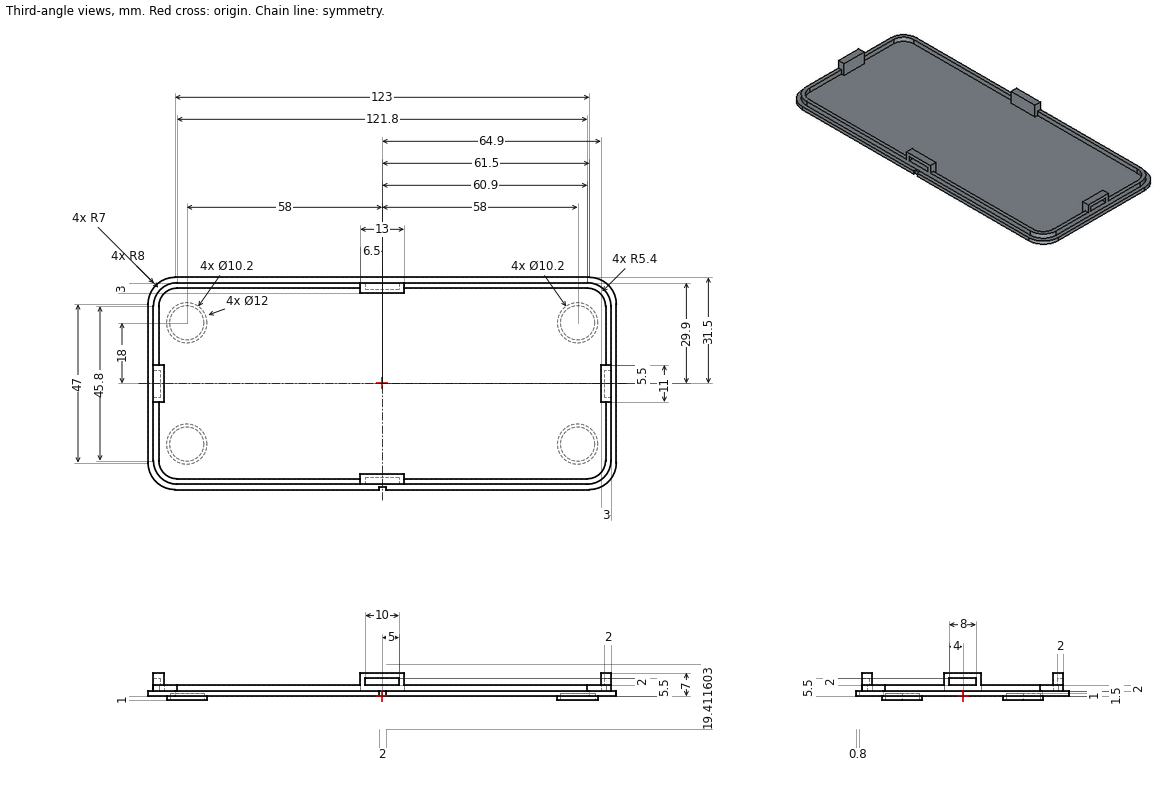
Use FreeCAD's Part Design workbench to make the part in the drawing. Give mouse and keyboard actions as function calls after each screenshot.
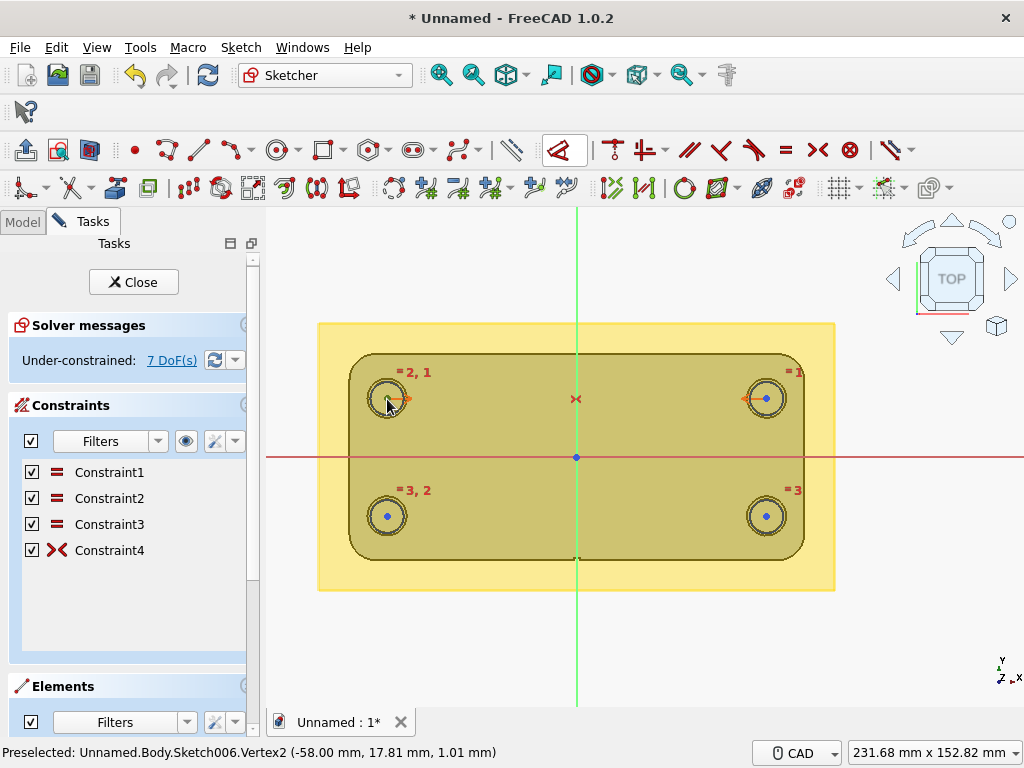
click(387, 517)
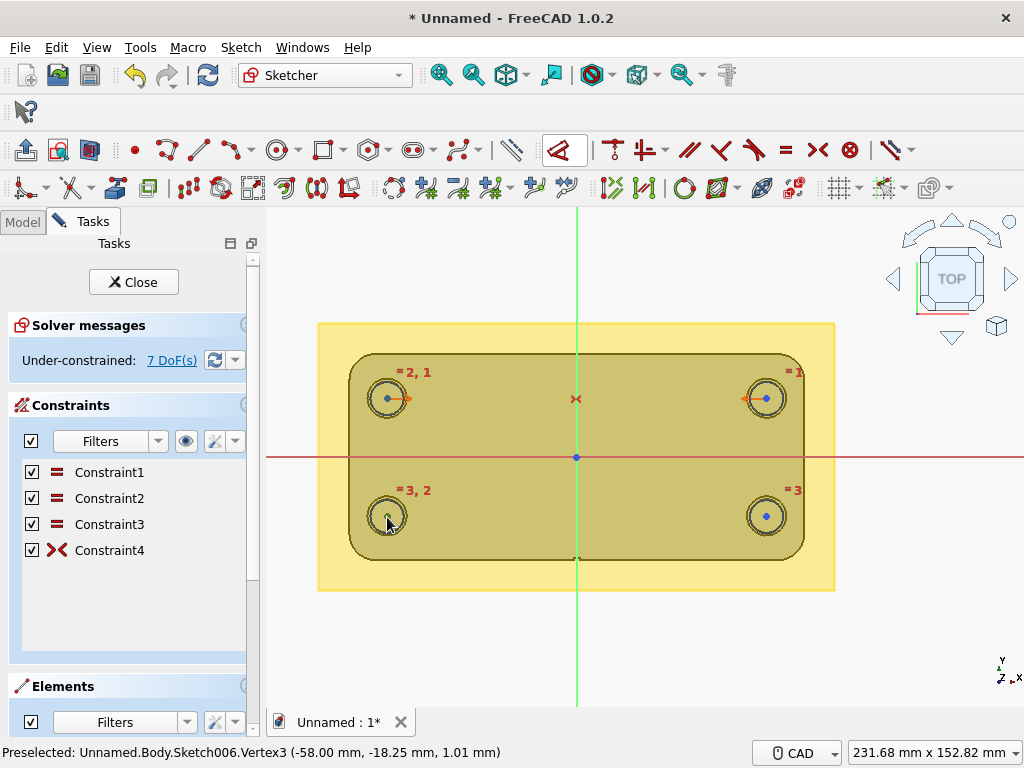
click(334, 457)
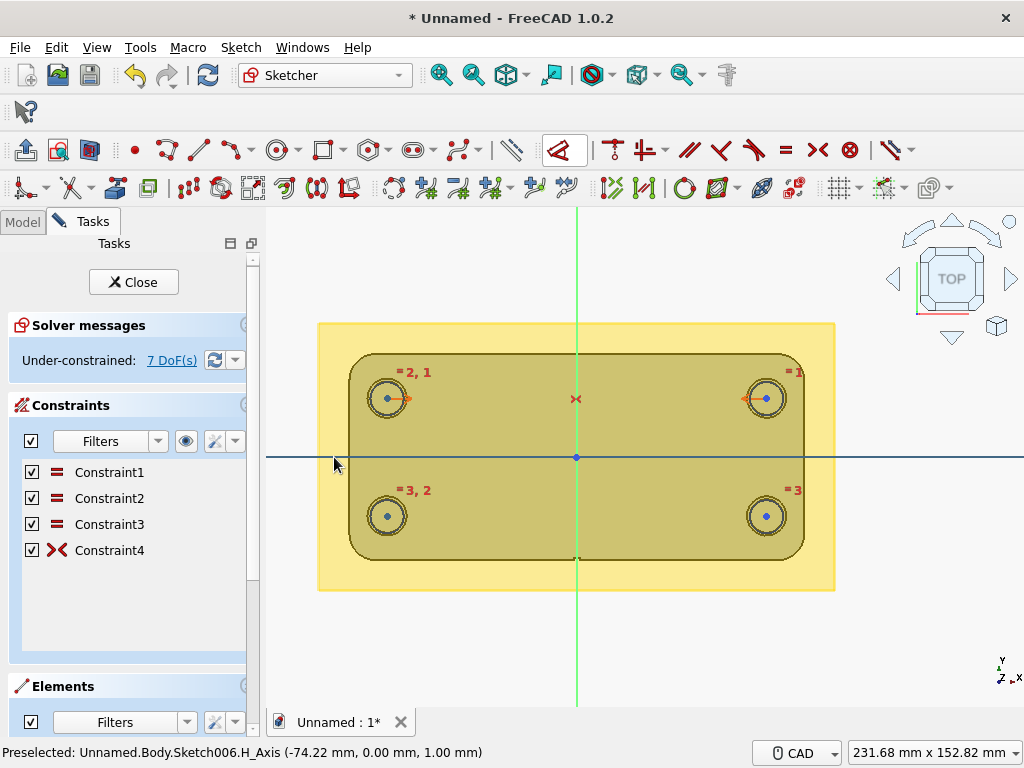
key(s)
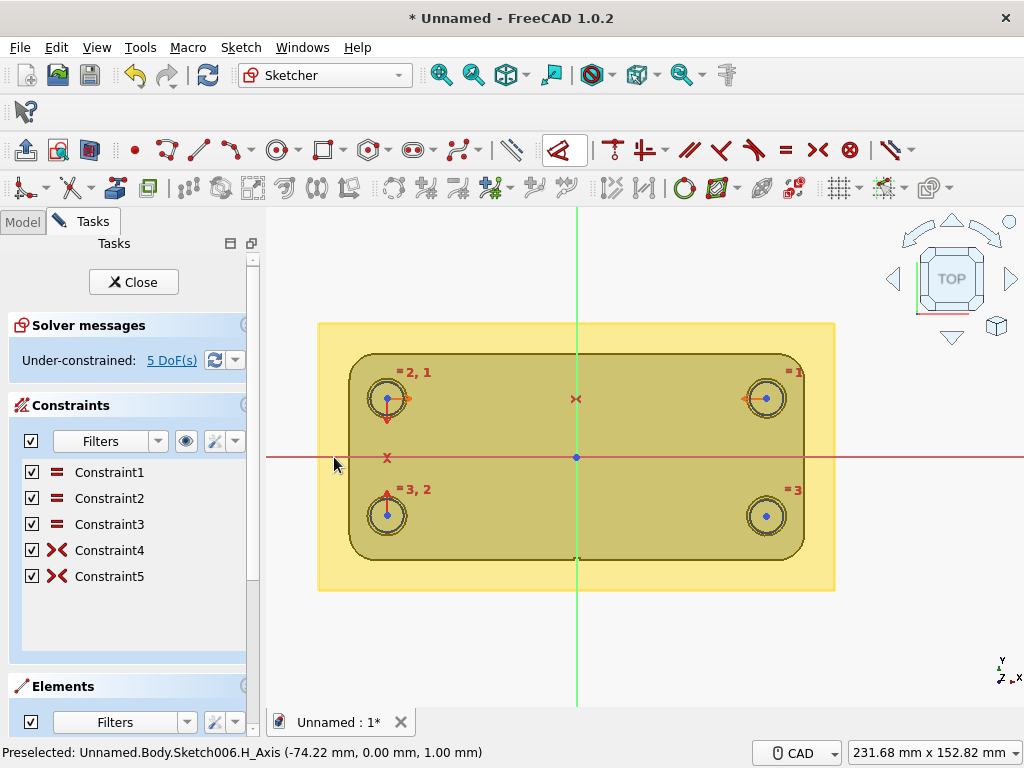
click(767, 399)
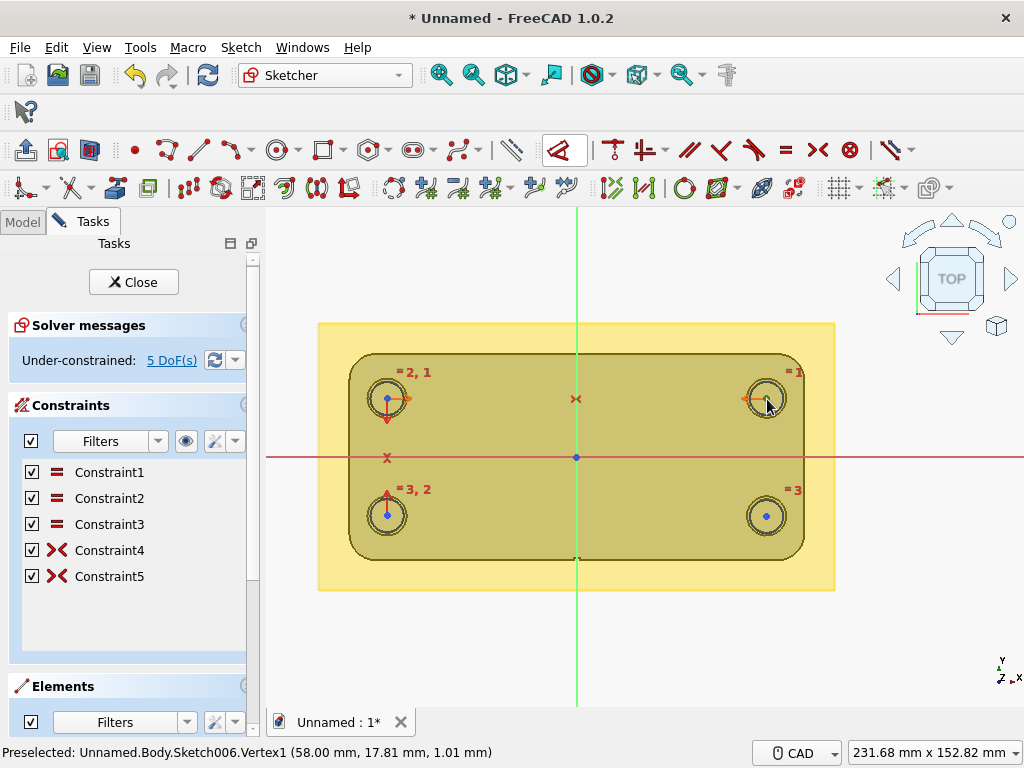
click(767, 517)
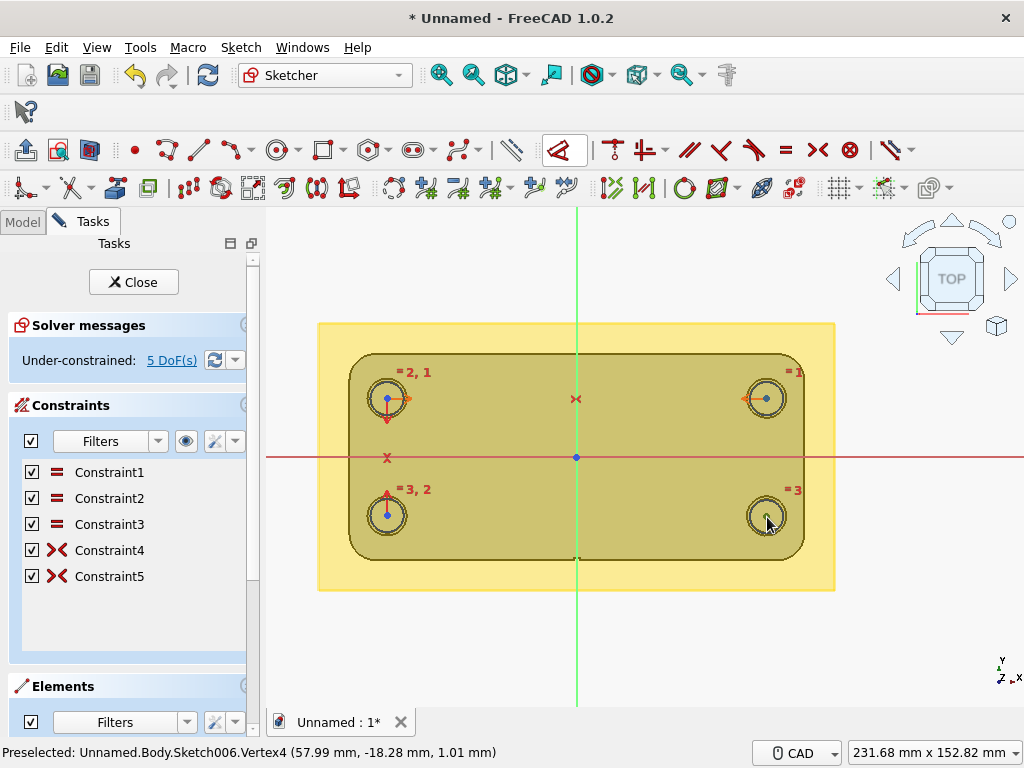
click(334, 457)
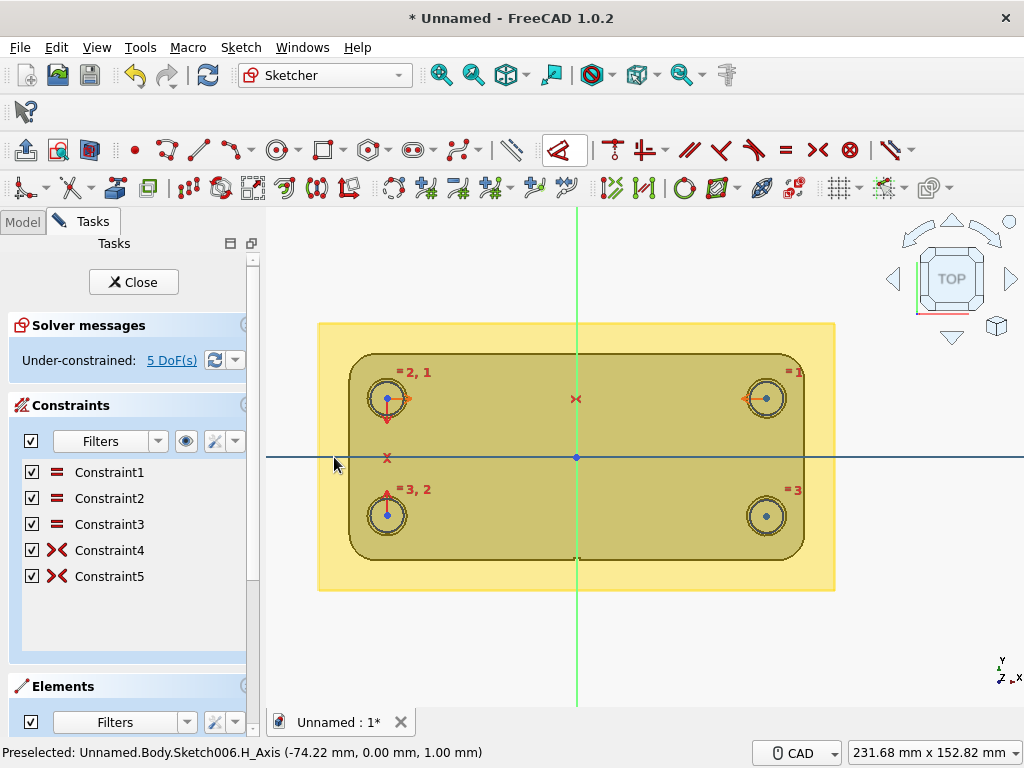
key(s)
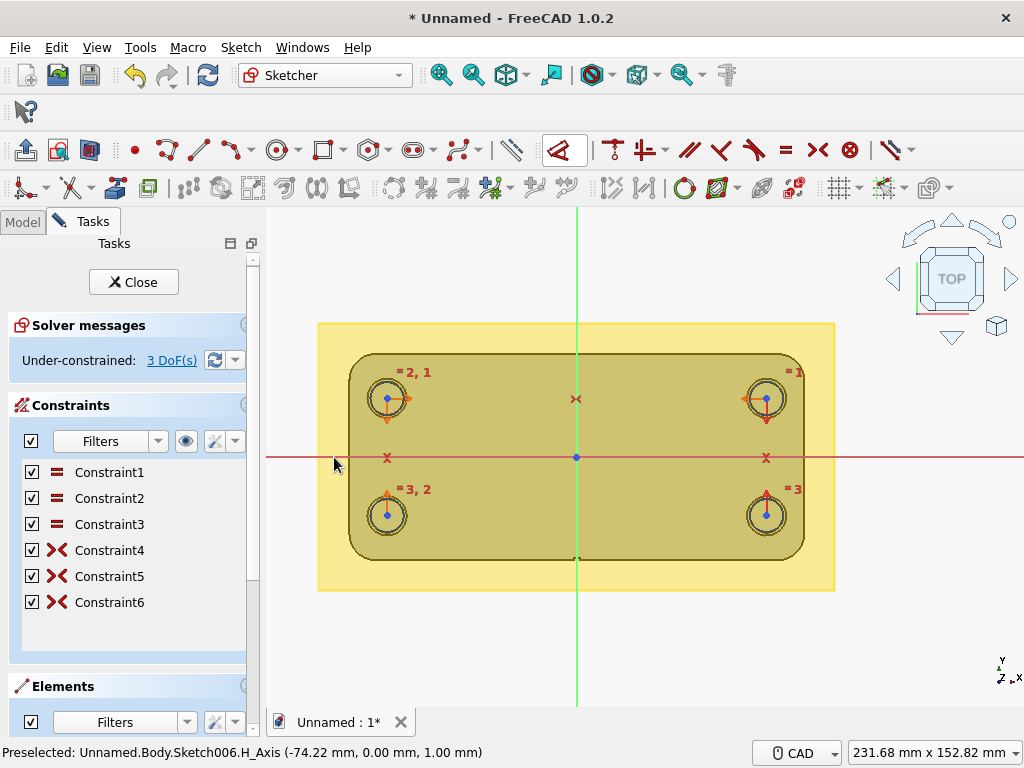
click(778, 387)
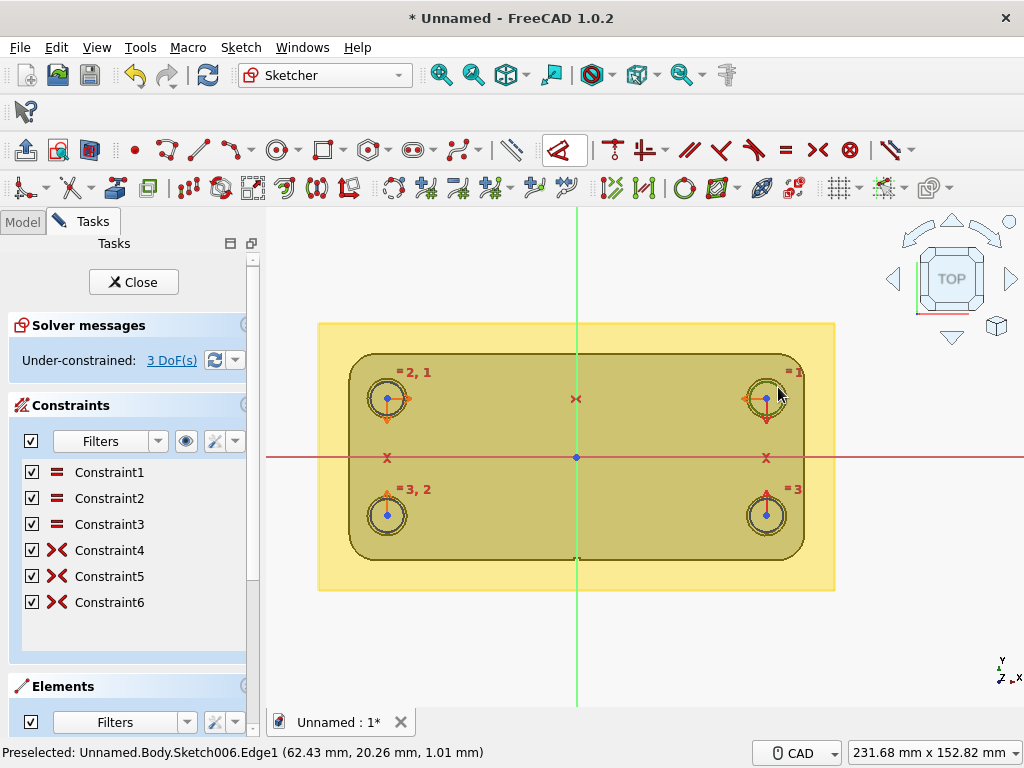
key(k)
key(o)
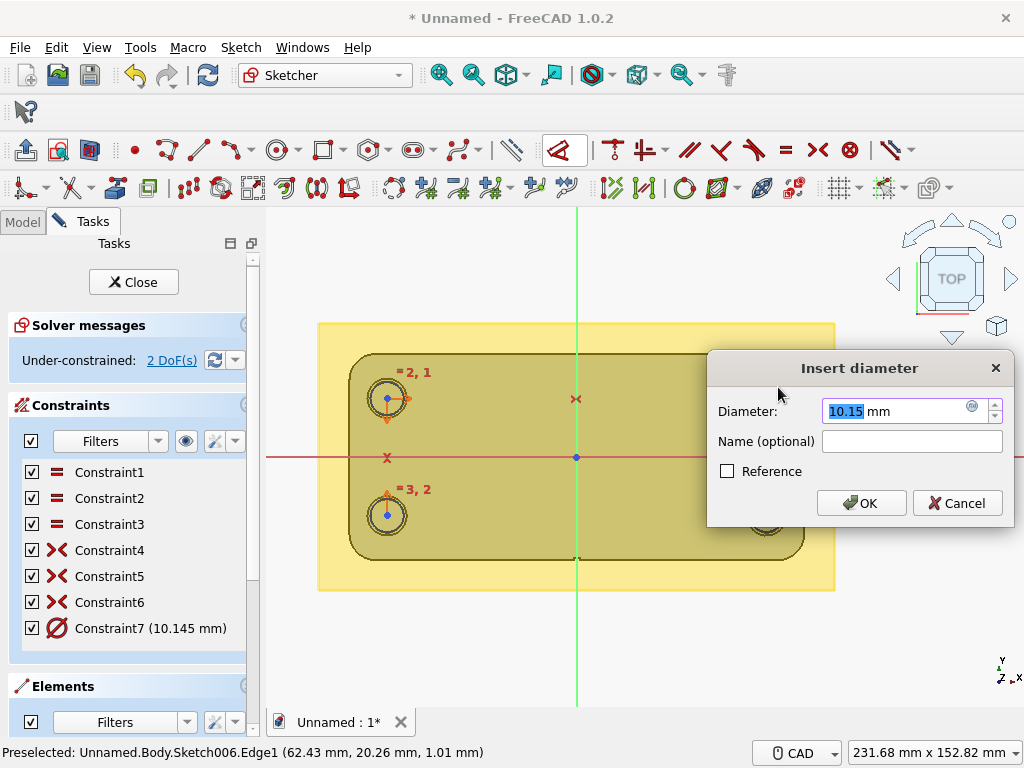
text(10.2)
key(Return)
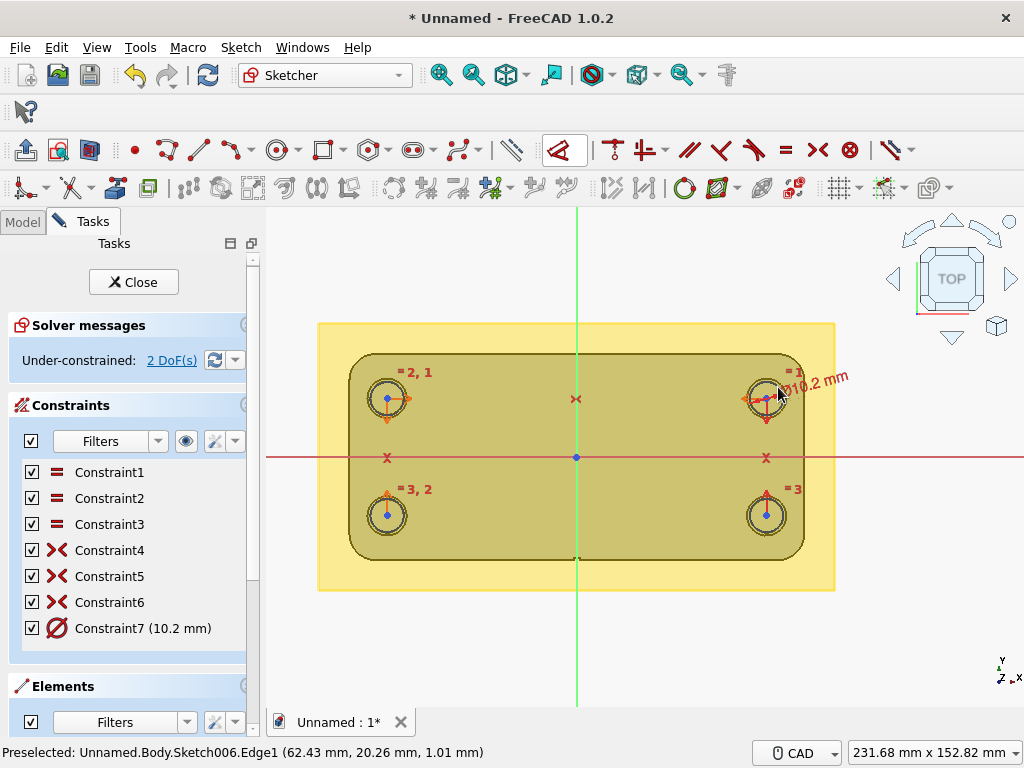
click(767, 399)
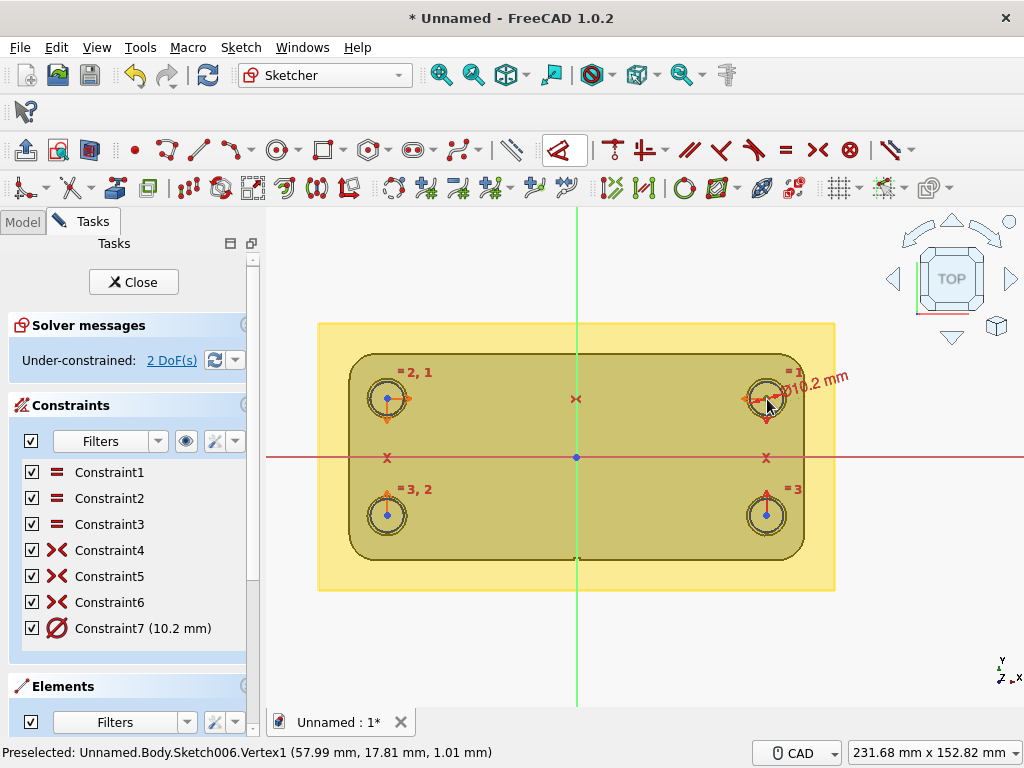
click(582, 150)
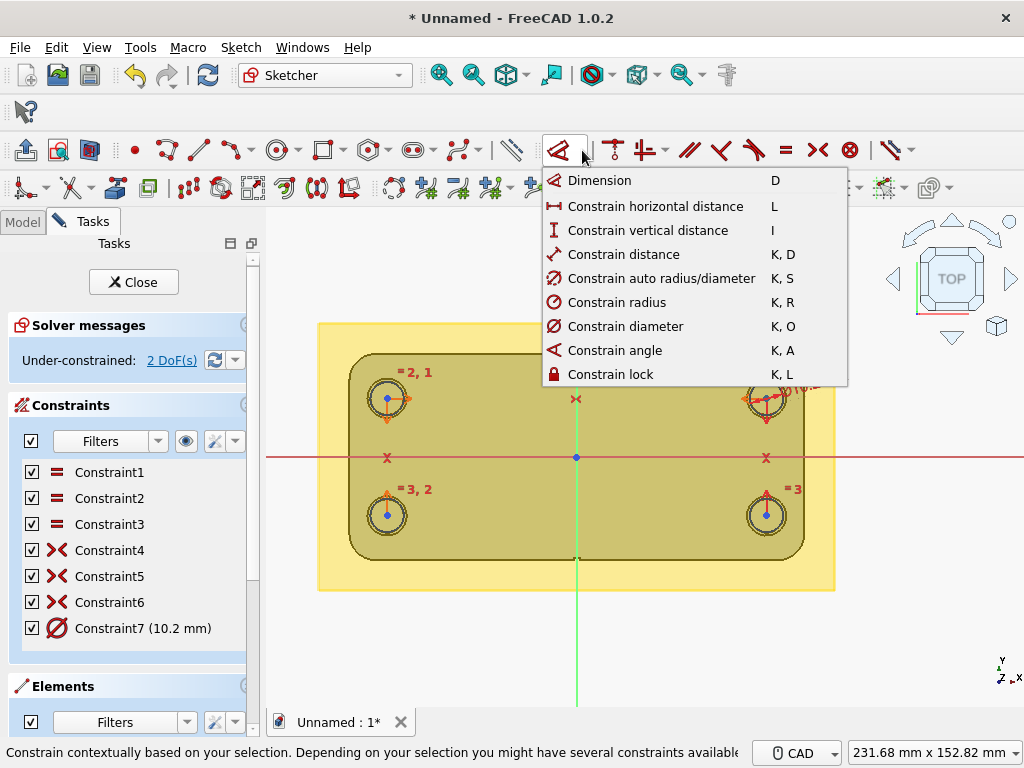
click(695, 206)